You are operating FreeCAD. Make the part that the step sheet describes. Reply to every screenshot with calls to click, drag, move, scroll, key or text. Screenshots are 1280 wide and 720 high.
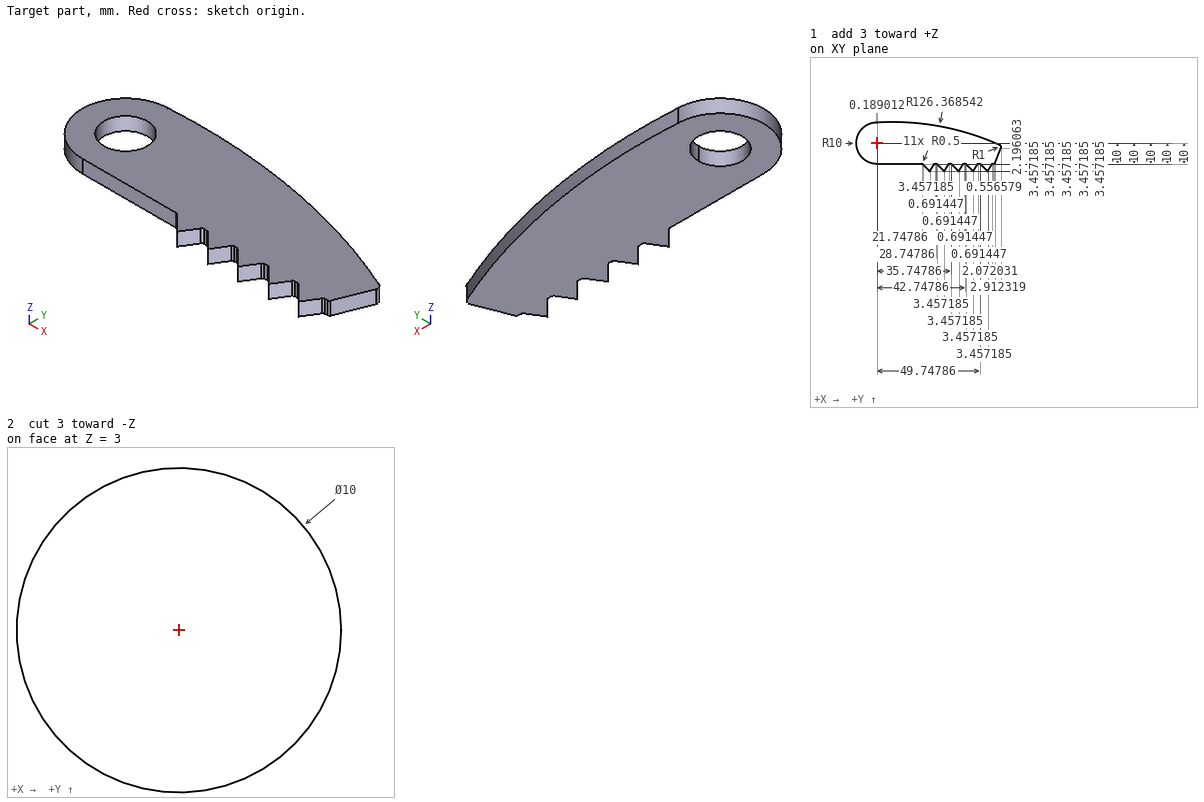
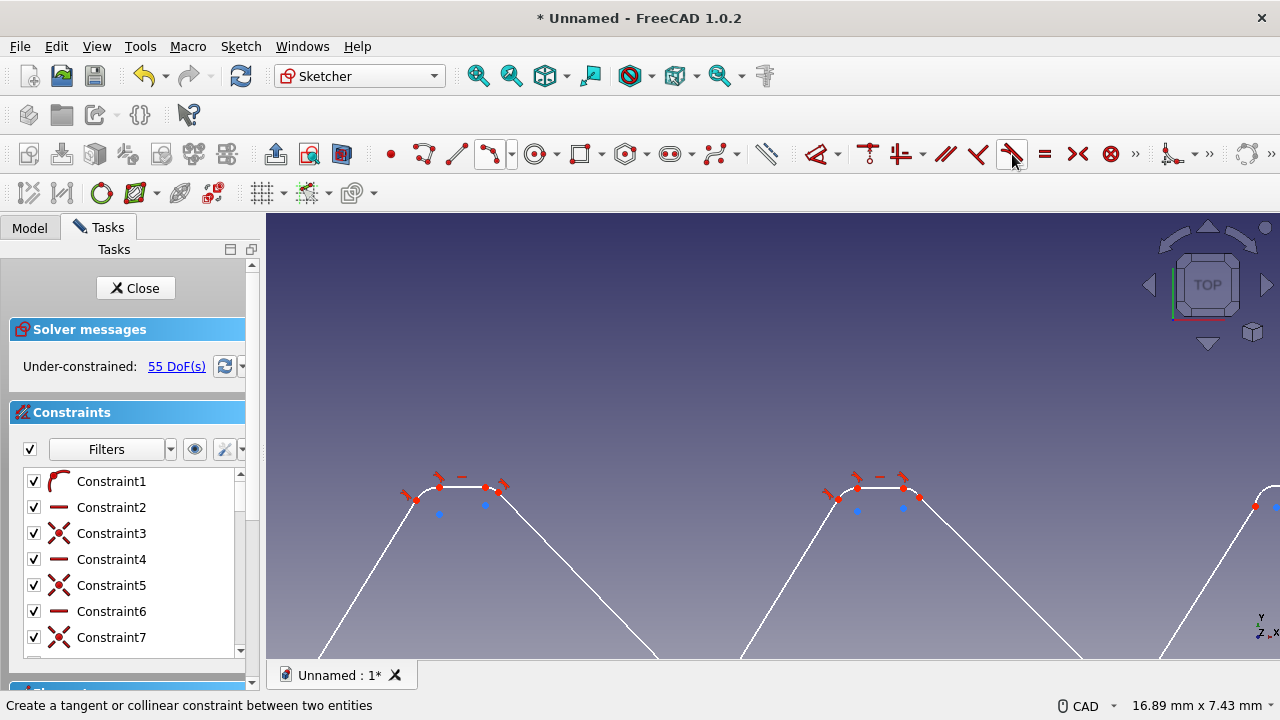
scroll(840, 505, down, 10)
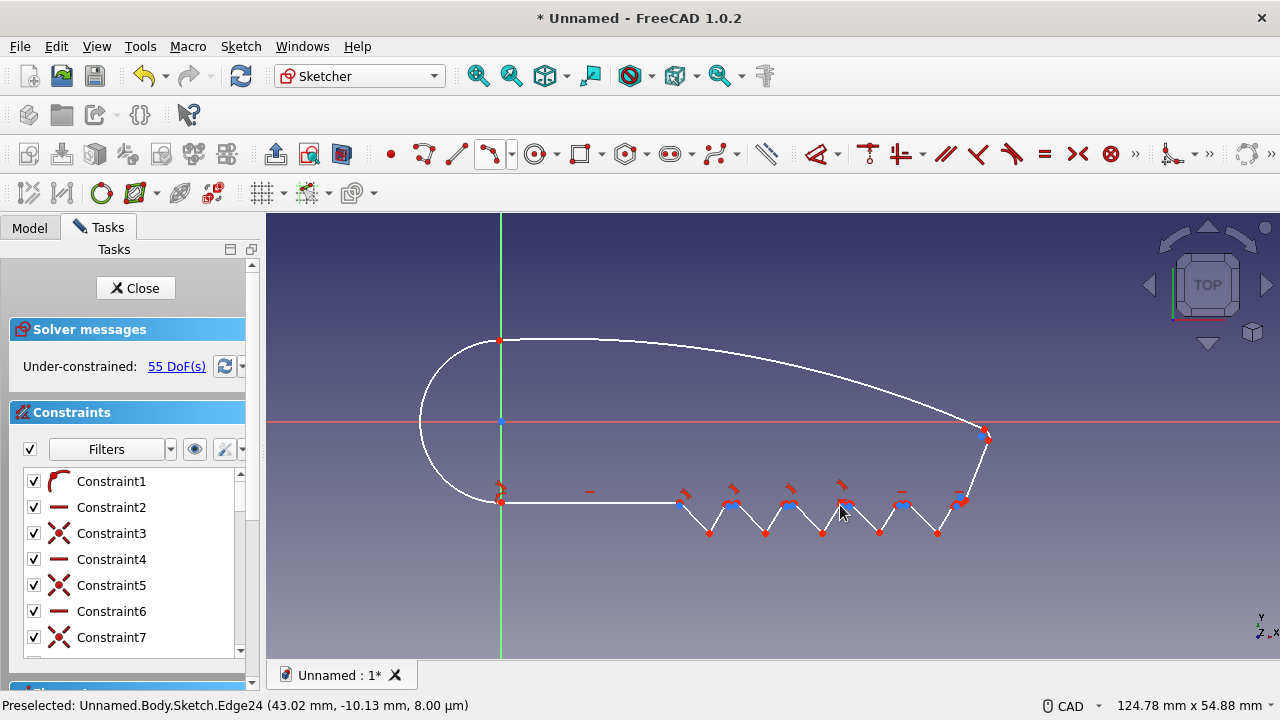
click(860, 513)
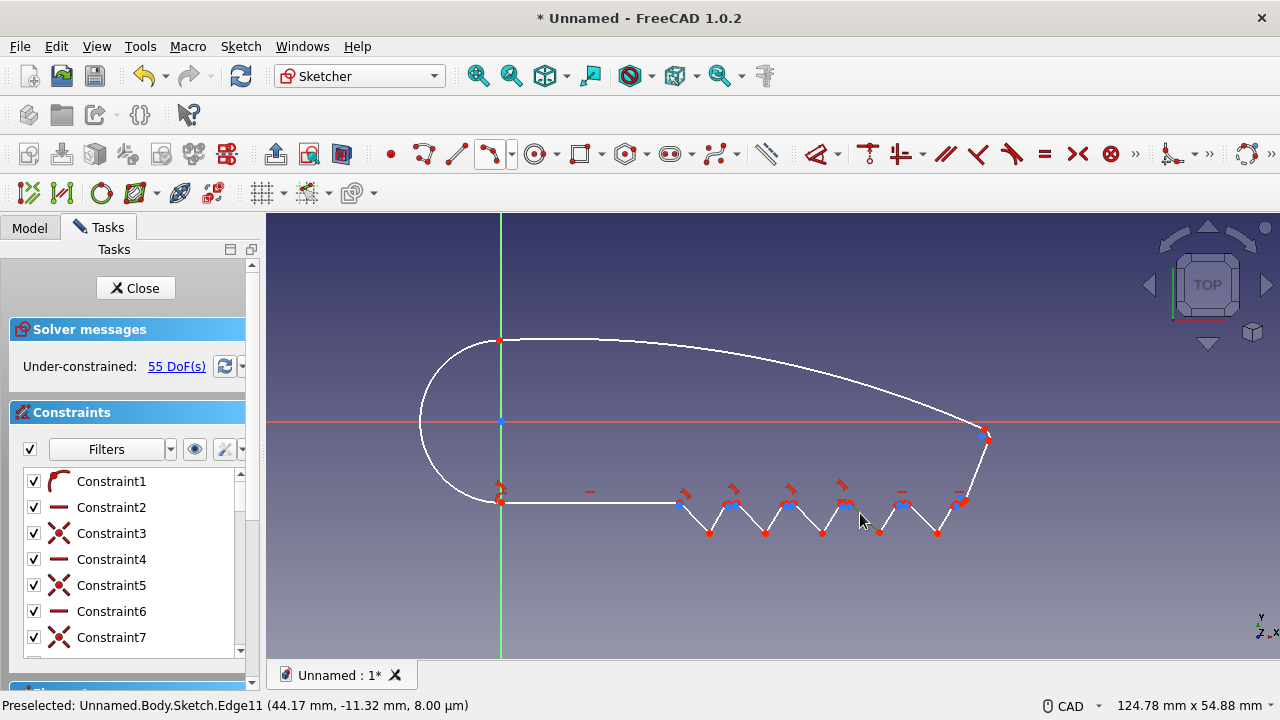
scroll(850, 504, up, 12)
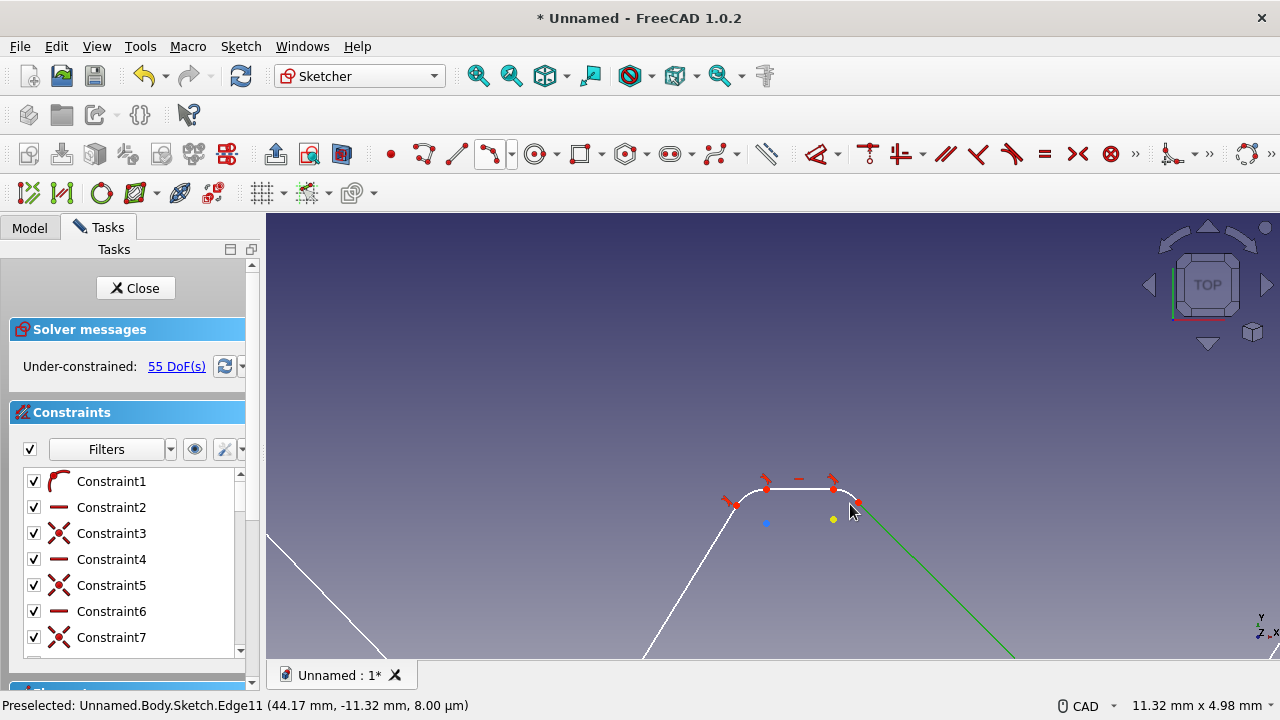
click(848, 493)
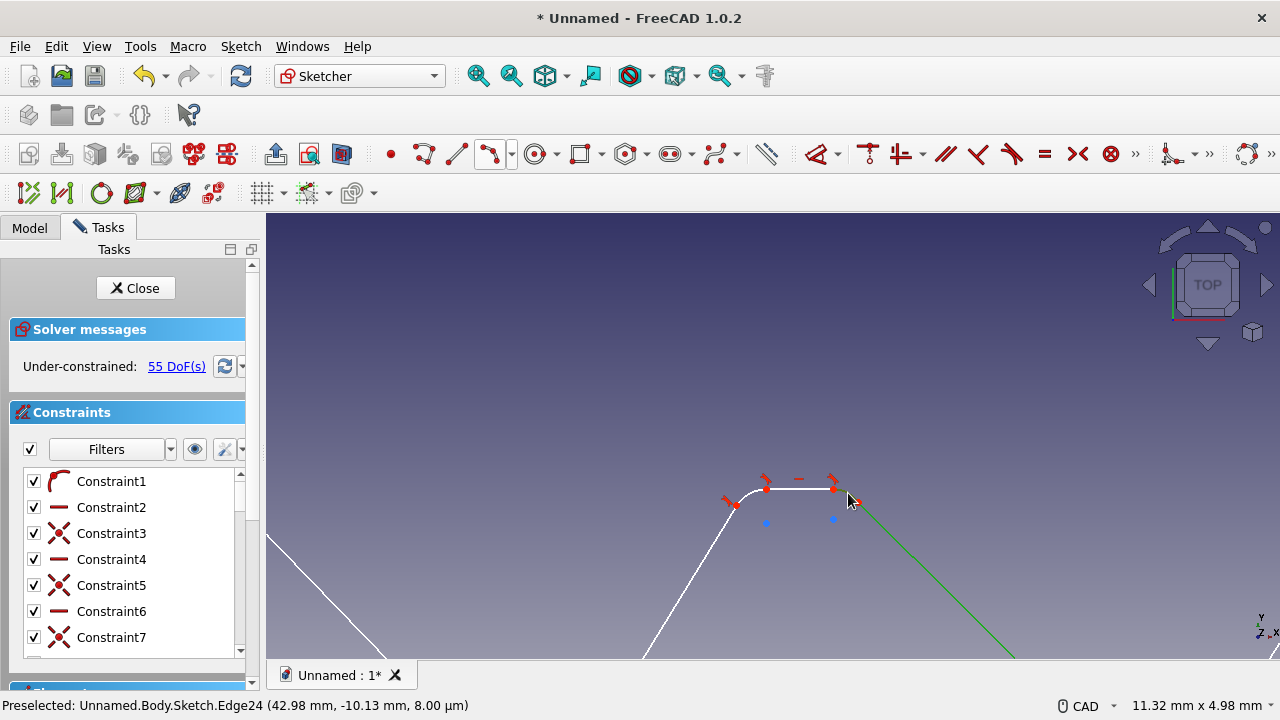
key(t)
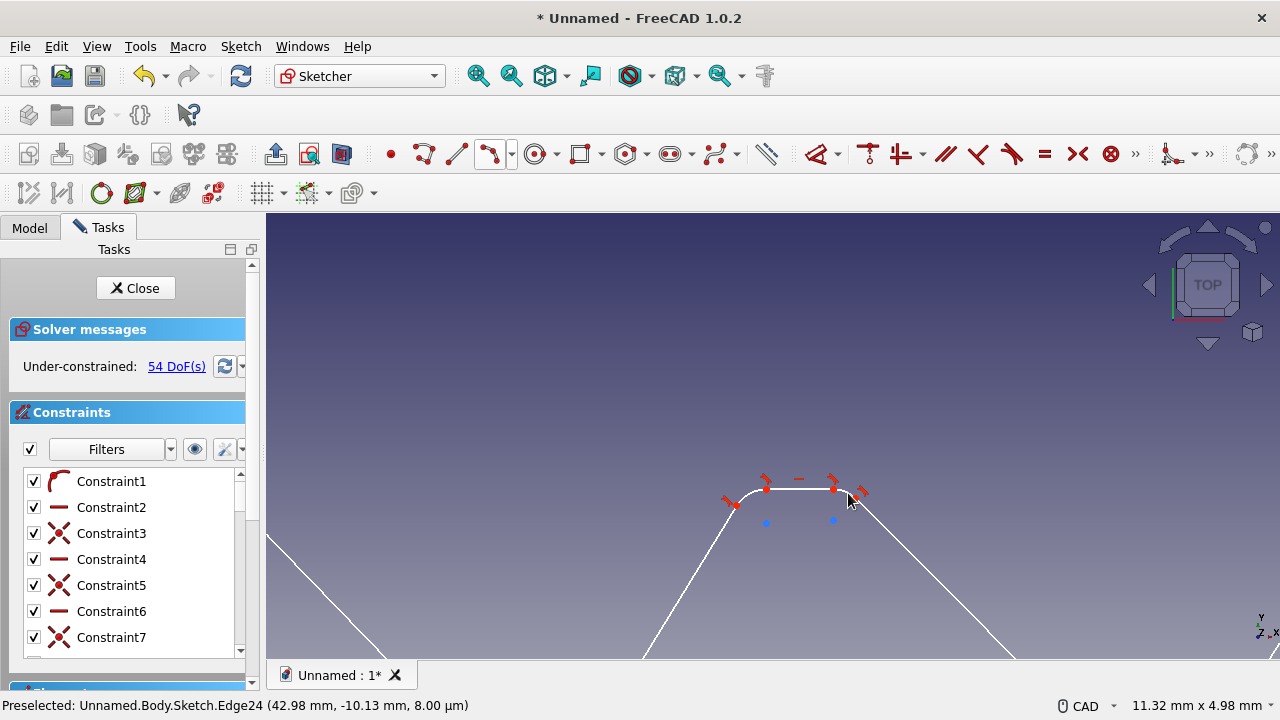
scroll(851, 504, down, 12)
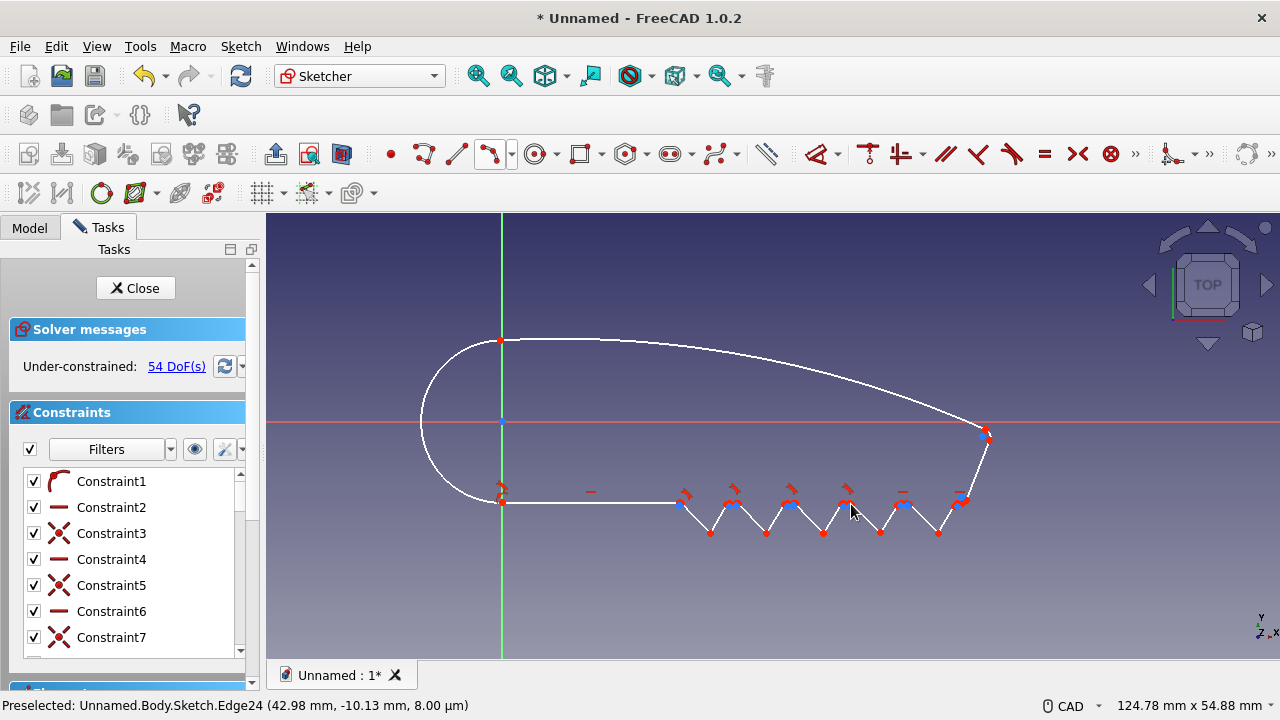
scroll(886, 525, up, 2)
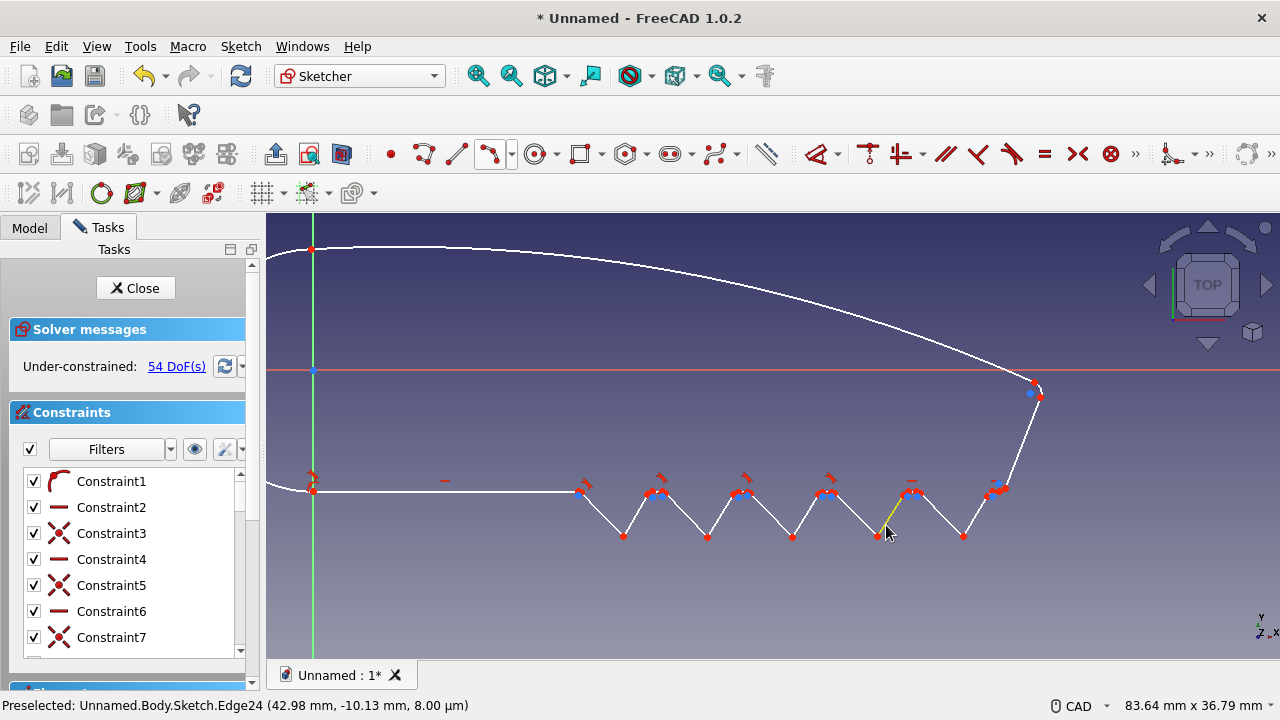
click(885, 524)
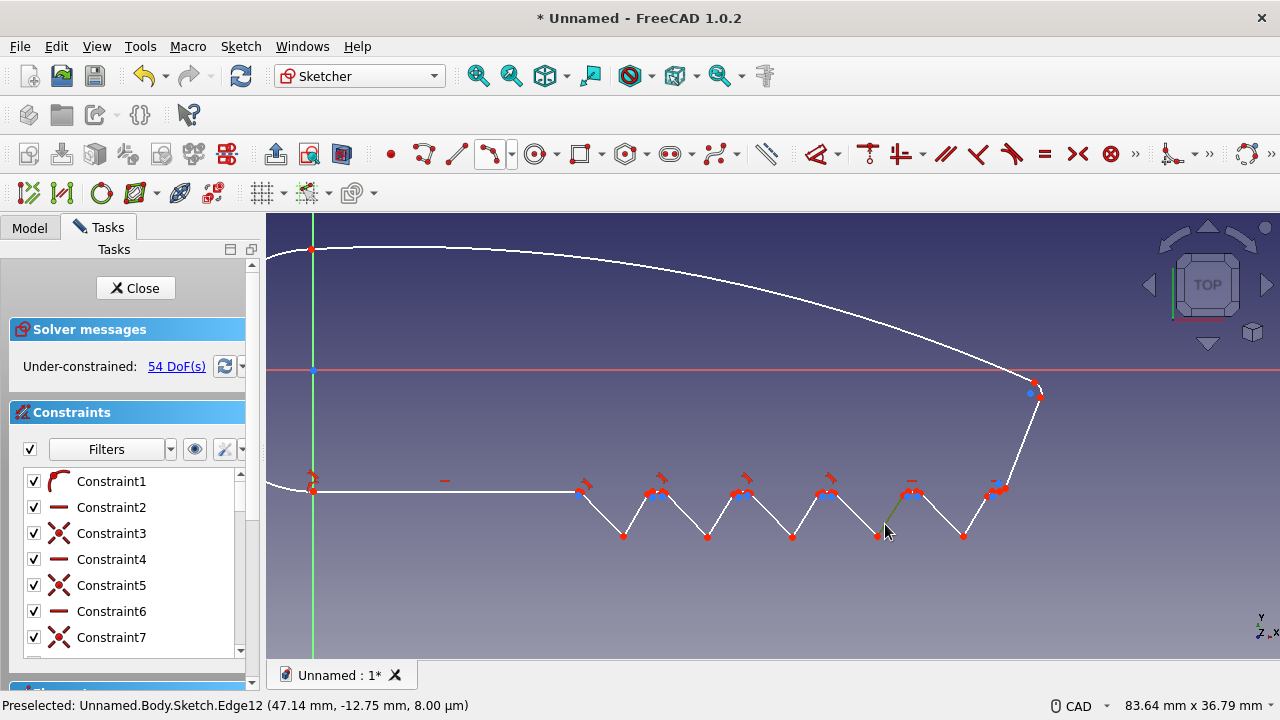
scroll(905, 493, up, 7)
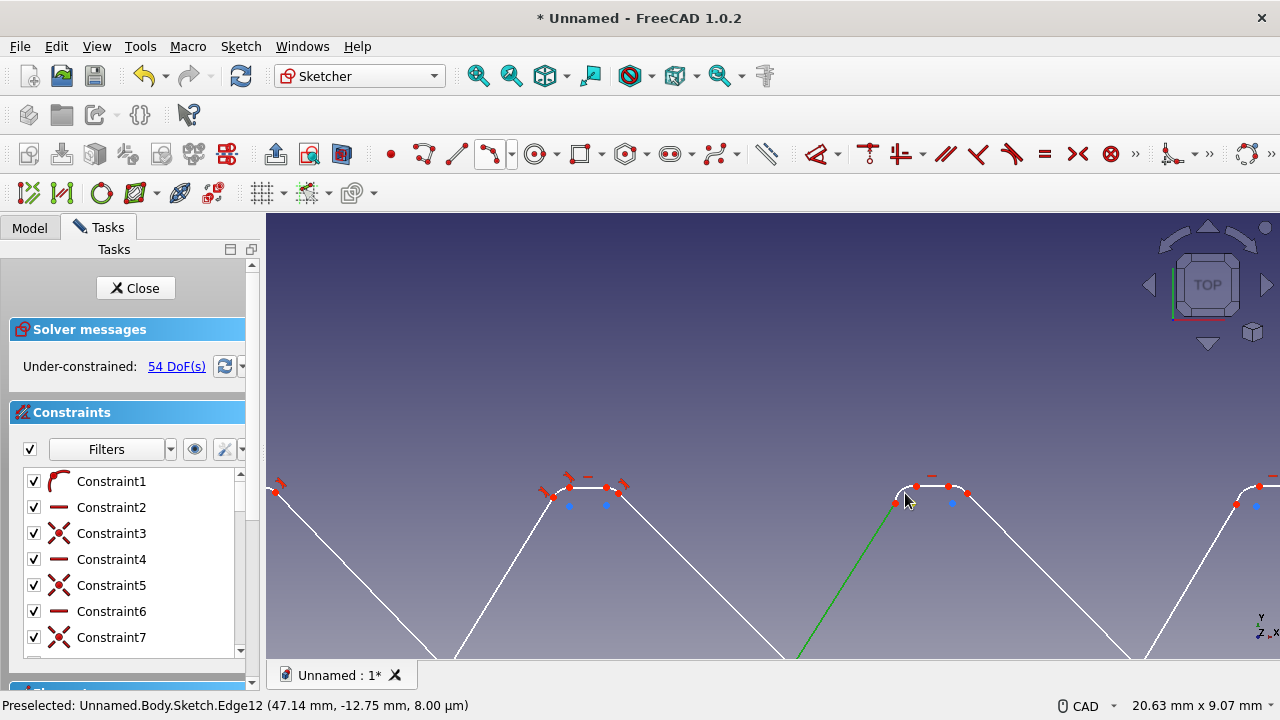
click(902, 490)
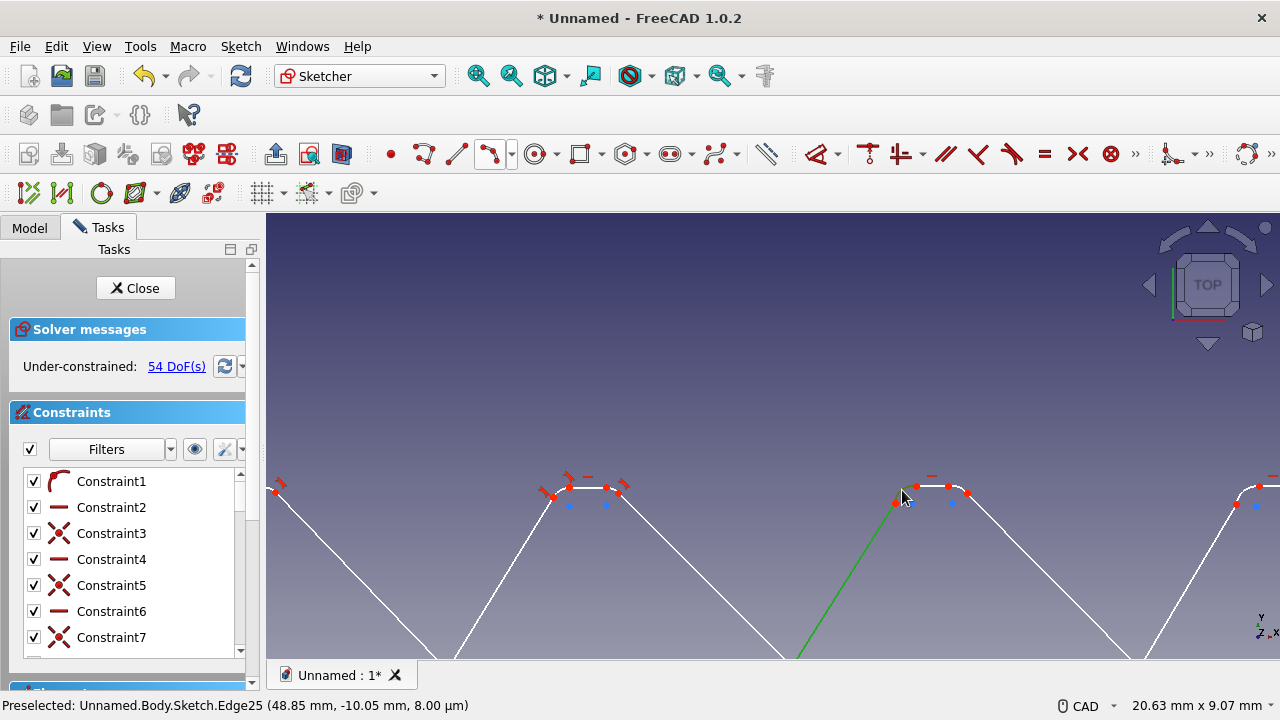
key(t)